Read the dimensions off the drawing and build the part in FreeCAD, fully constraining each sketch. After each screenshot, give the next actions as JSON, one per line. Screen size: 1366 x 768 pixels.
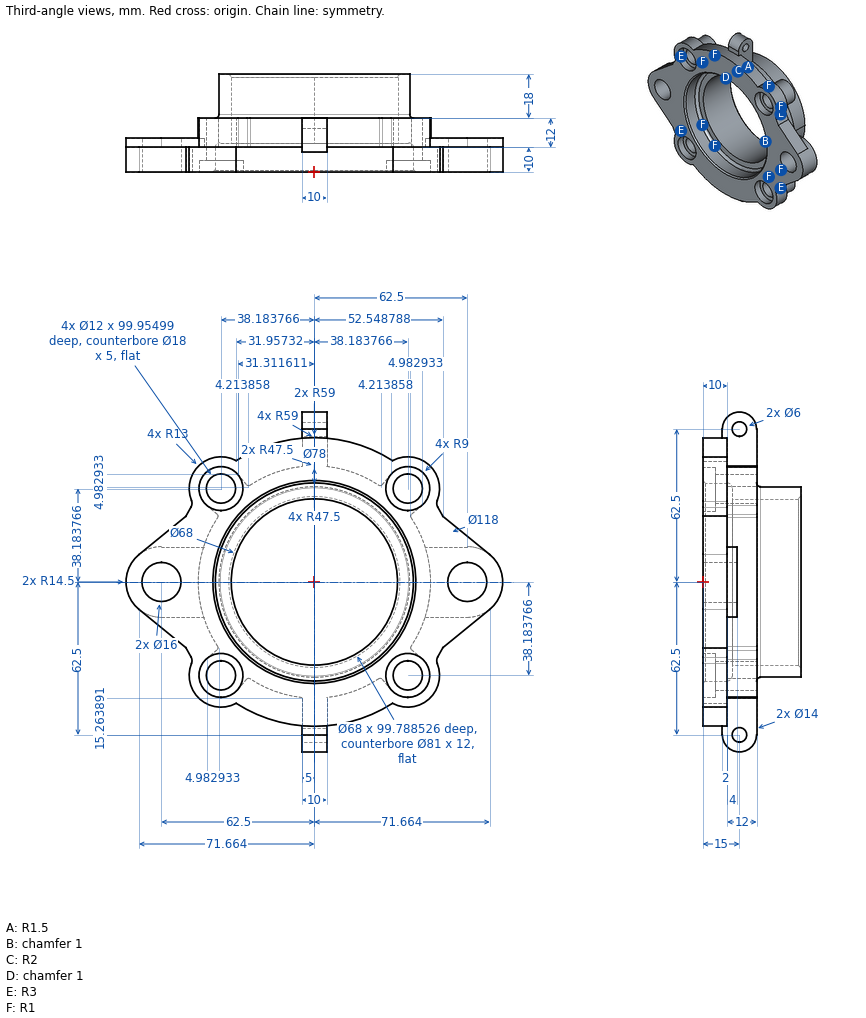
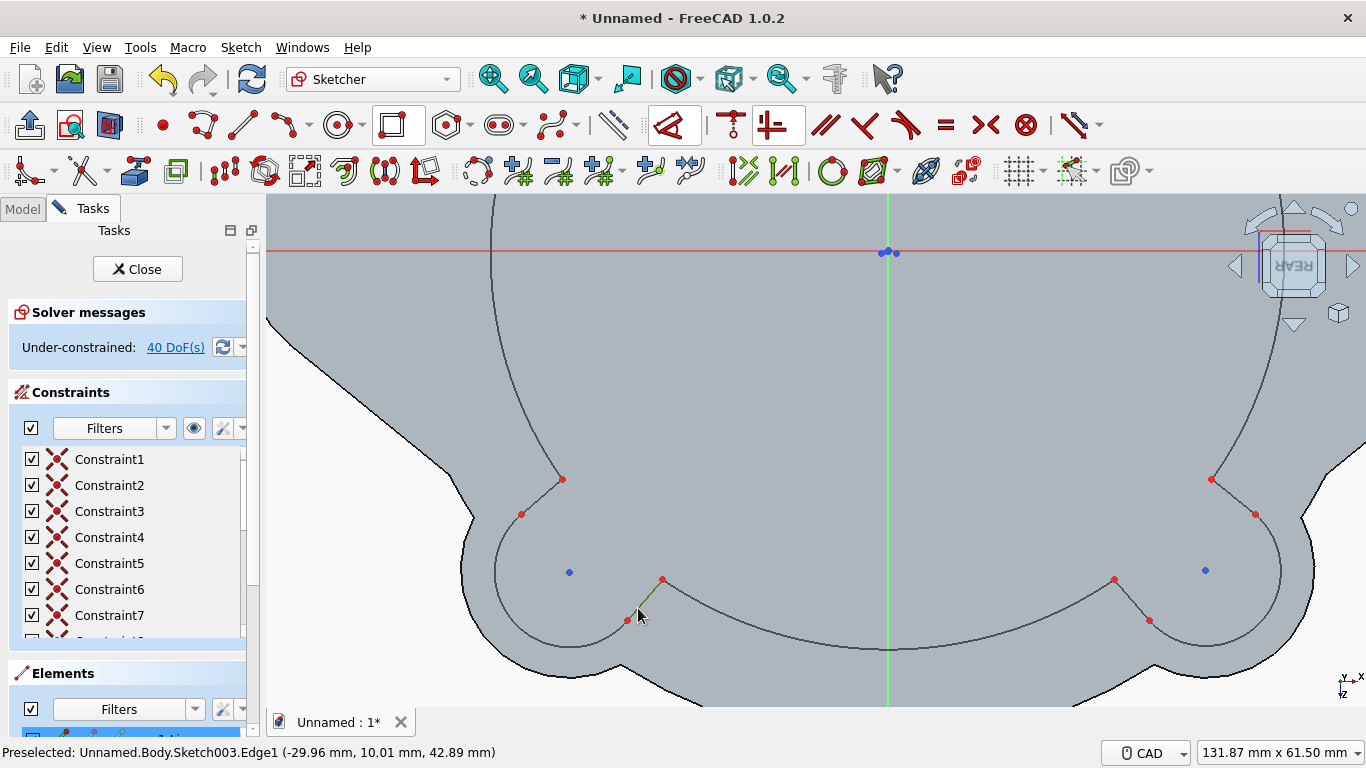
{"action": "left_click", "coordinate": [495, 581]}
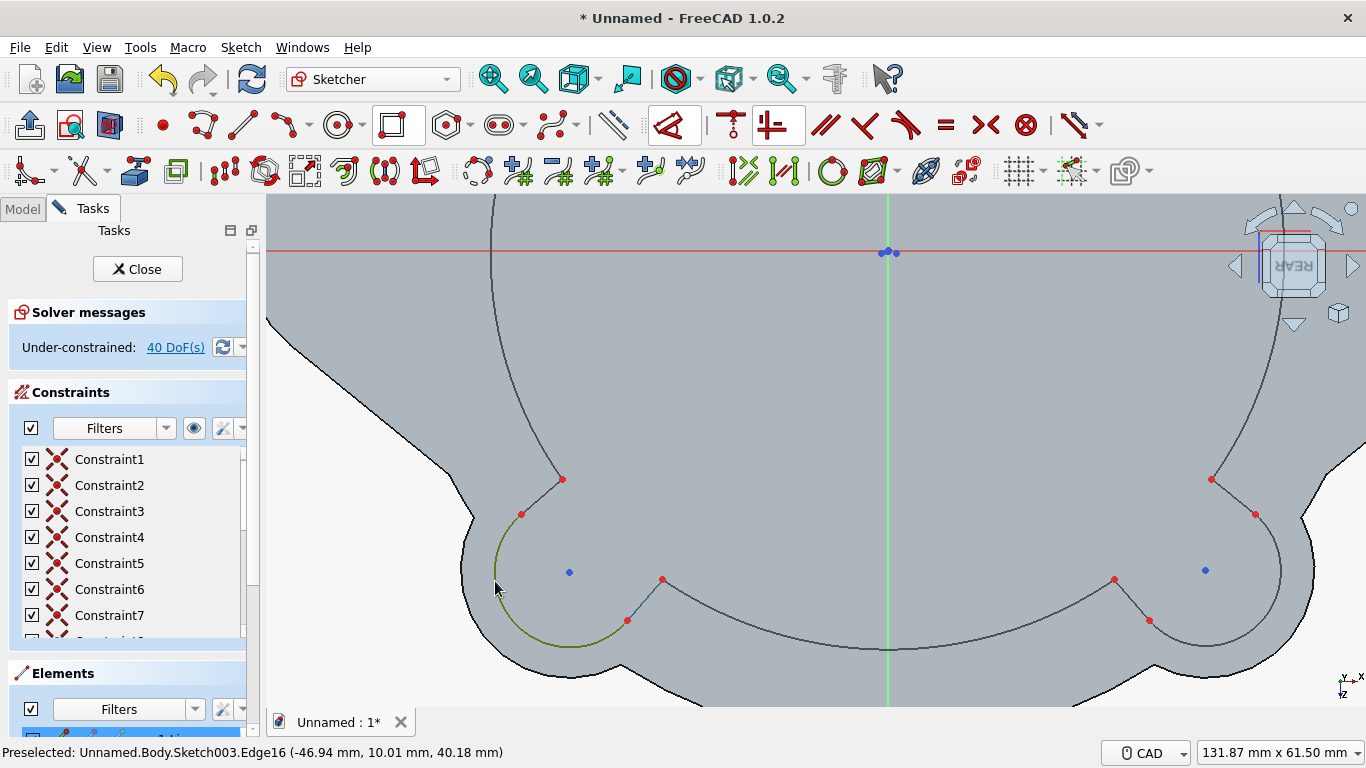
{"action": "left_click", "coordinate": [906, 126]}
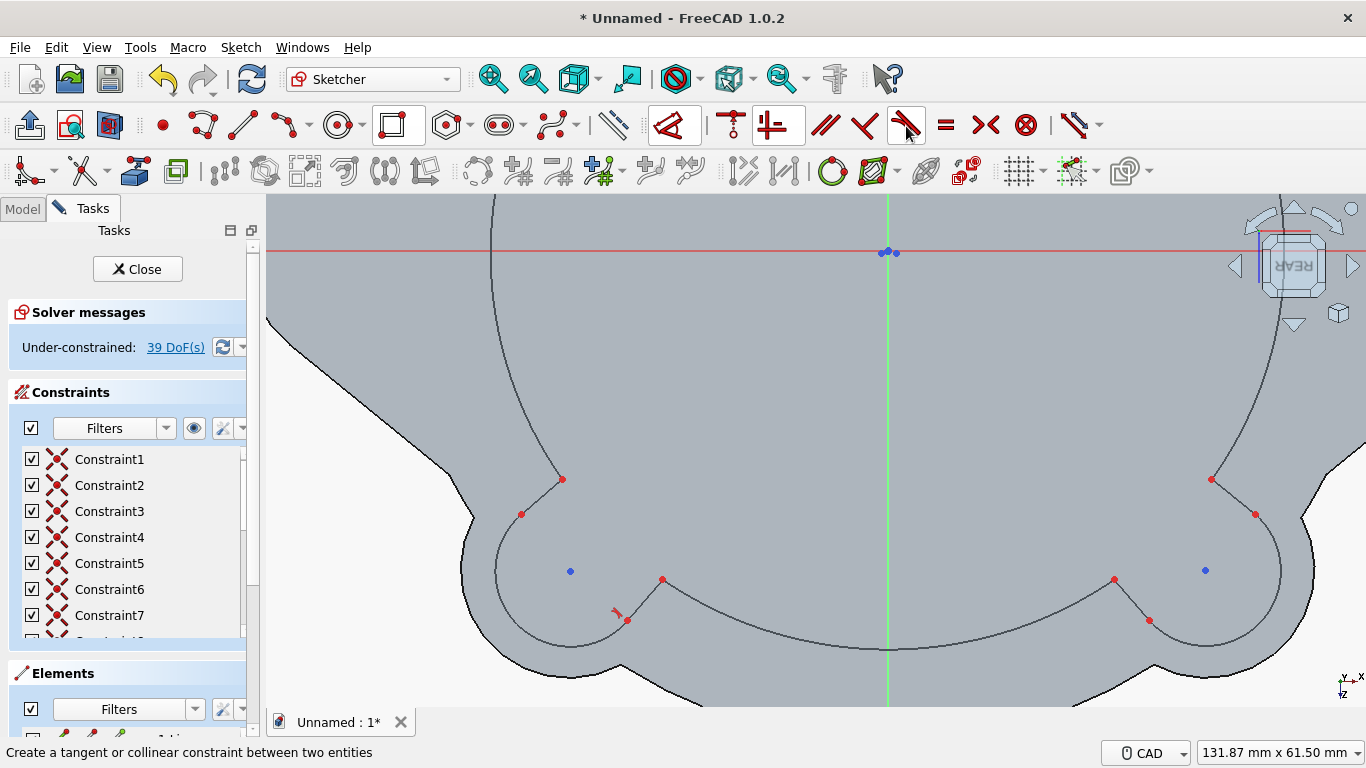
{"action": "left_click", "coordinate": [1125, 592]}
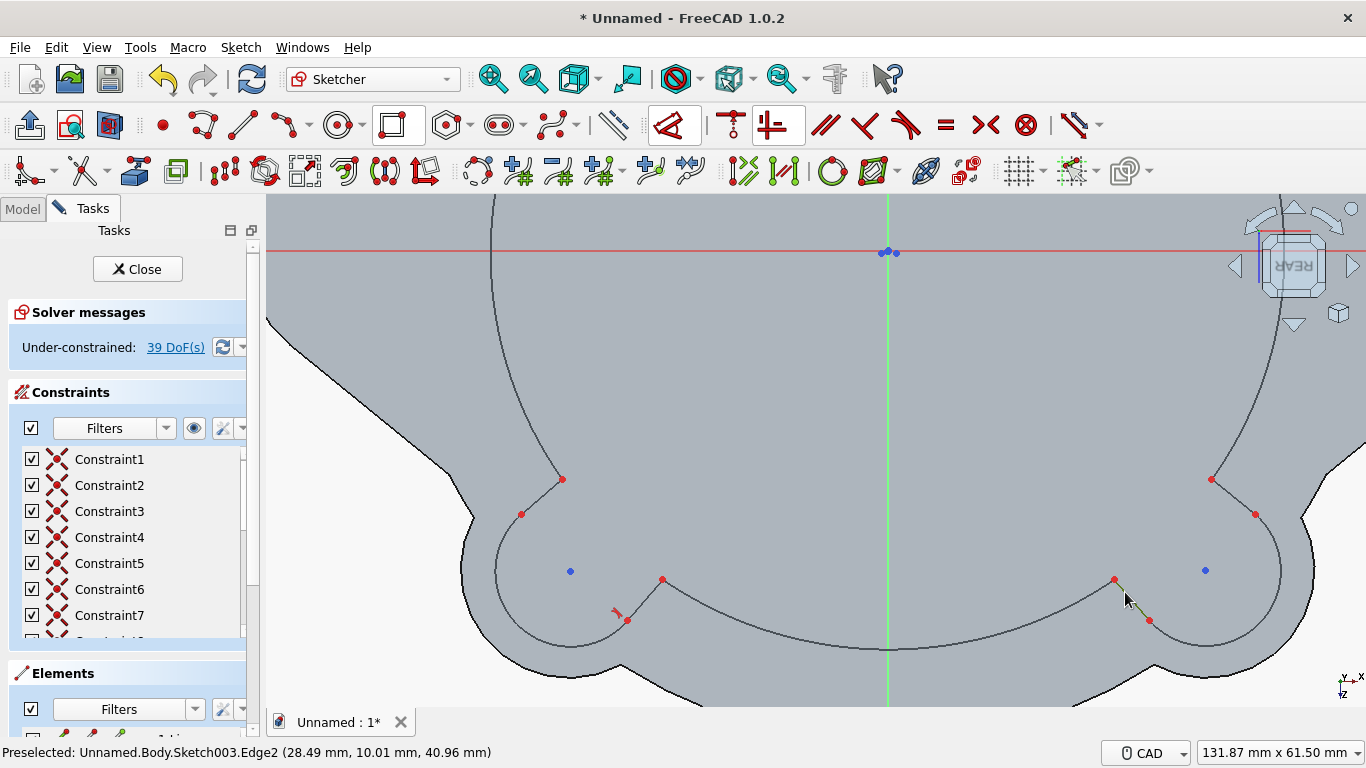
{"action": "left_click", "coordinate": [1191, 645]}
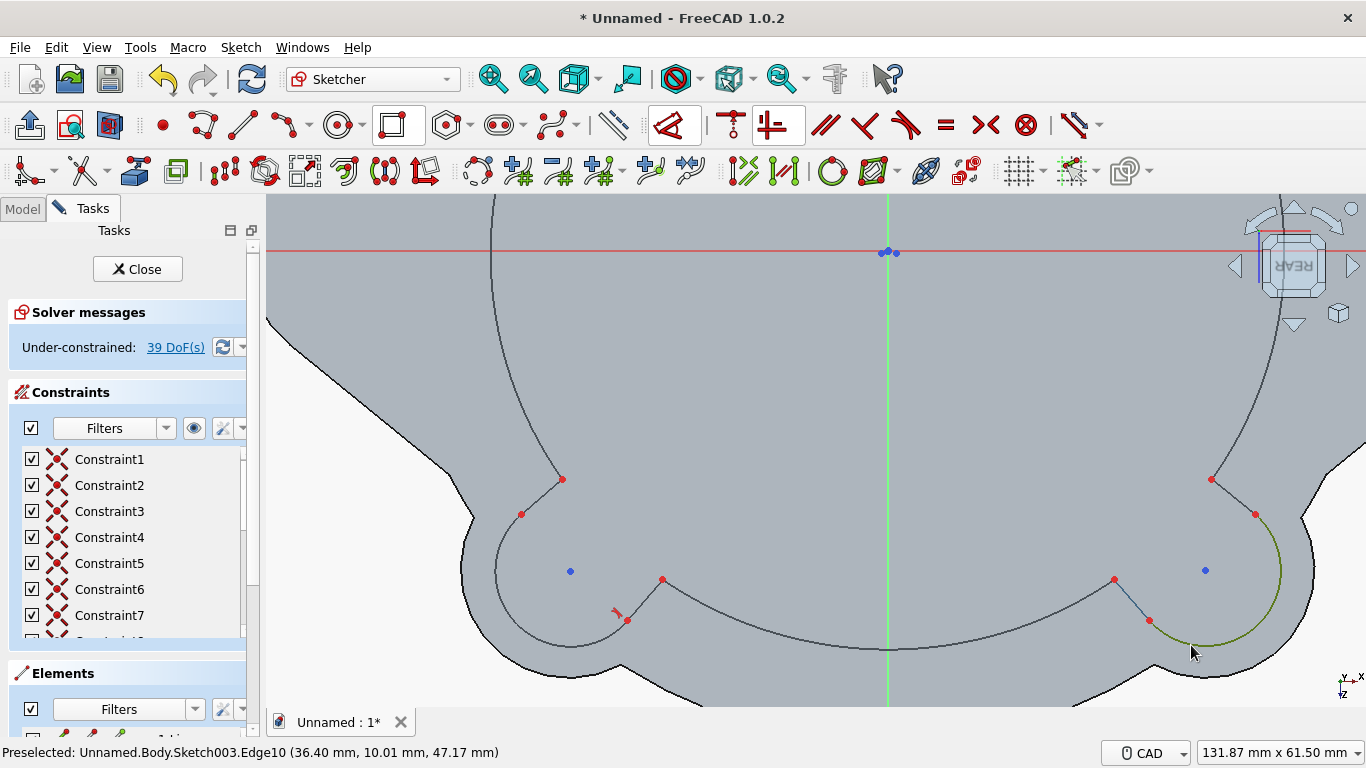
{"action": "left_click", "coordinate": [906, 126]}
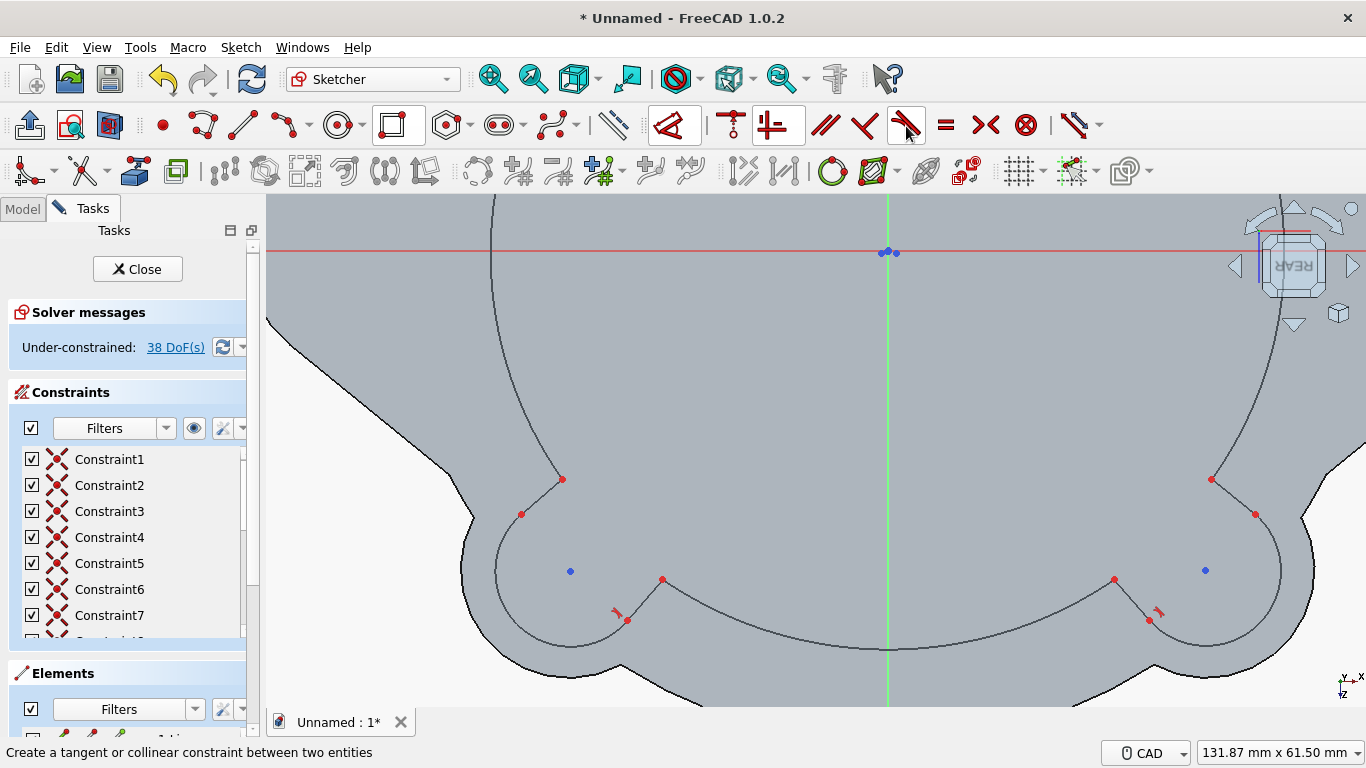
{"action": "scroll", "coordinate": [633, 613], "scroll_direction": "down", "scroll_amount": 4}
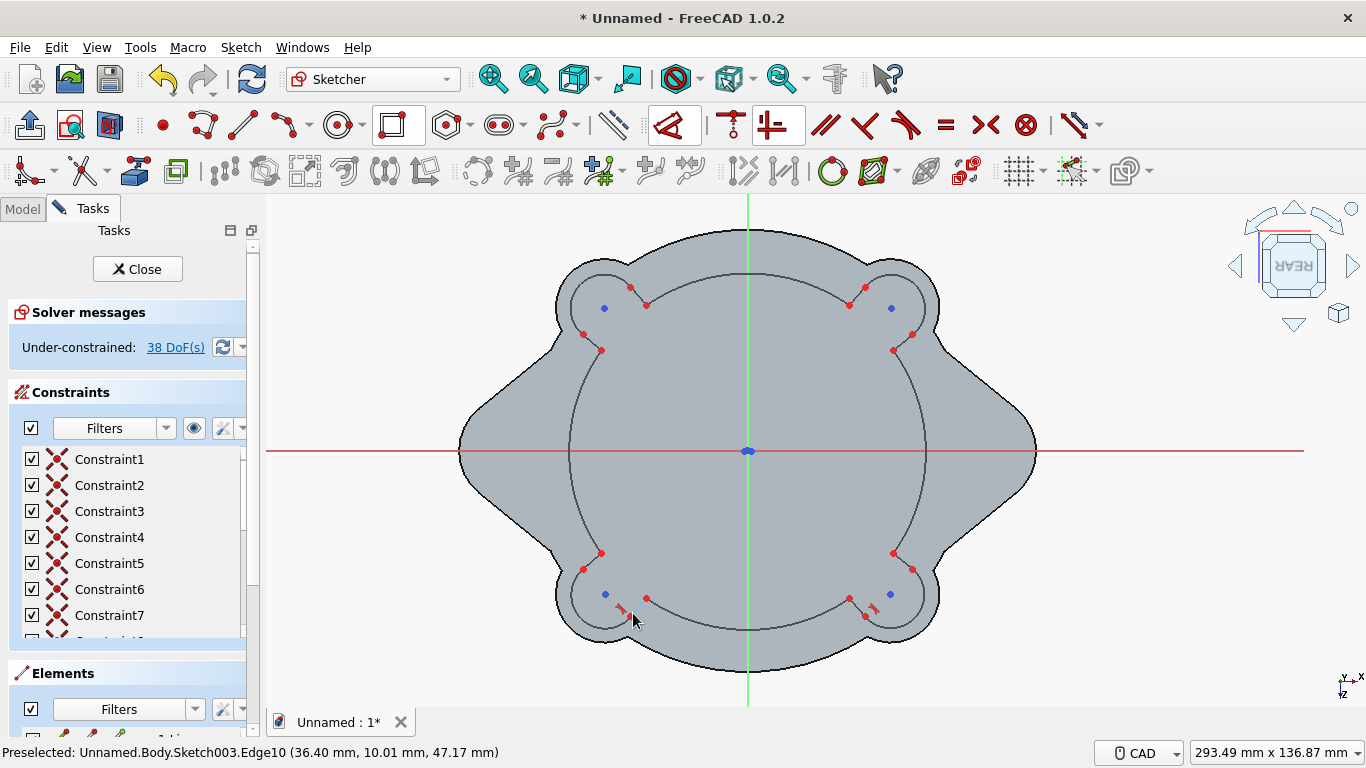
{"action": "scroll", "coordinate": [907, 564], "scroll_direction": "up", "scroll_amount": 4}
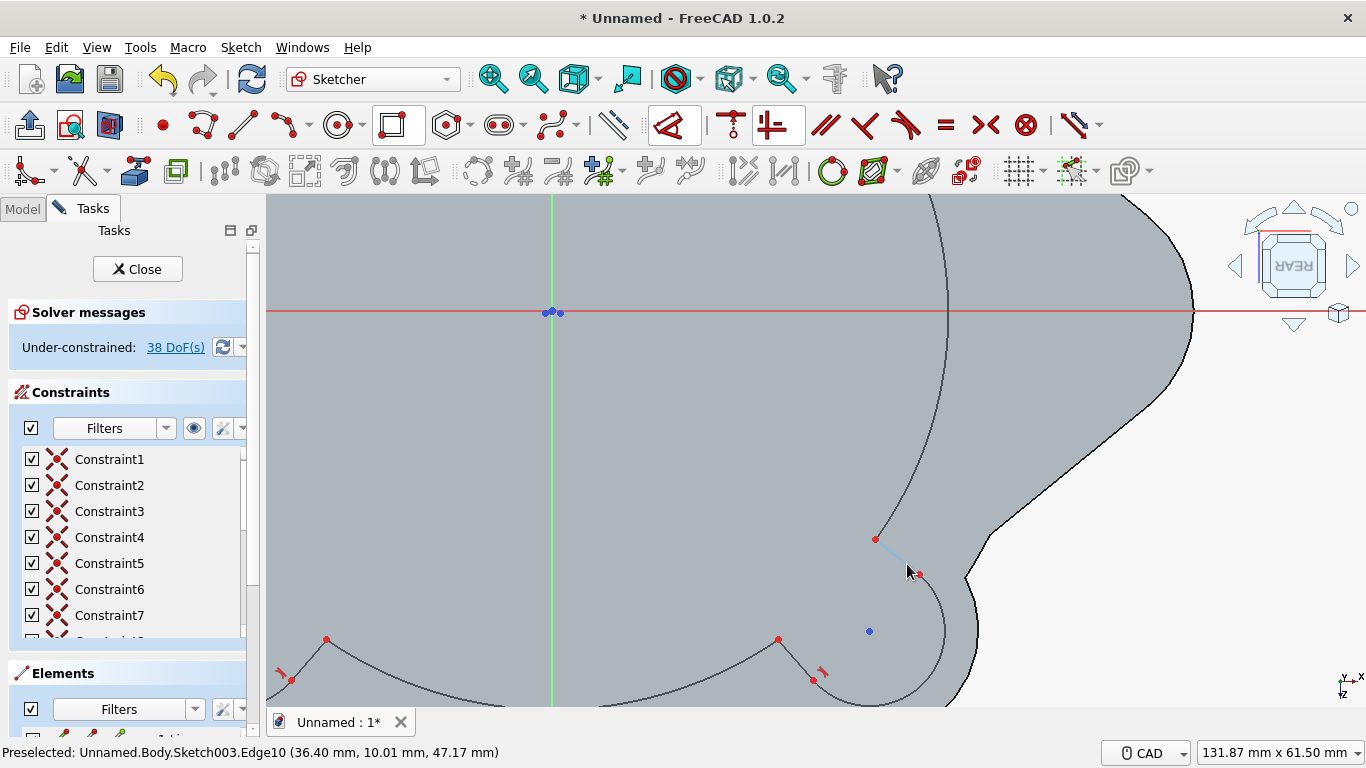
{"action": "left_click", "coordinate": [906, 564]}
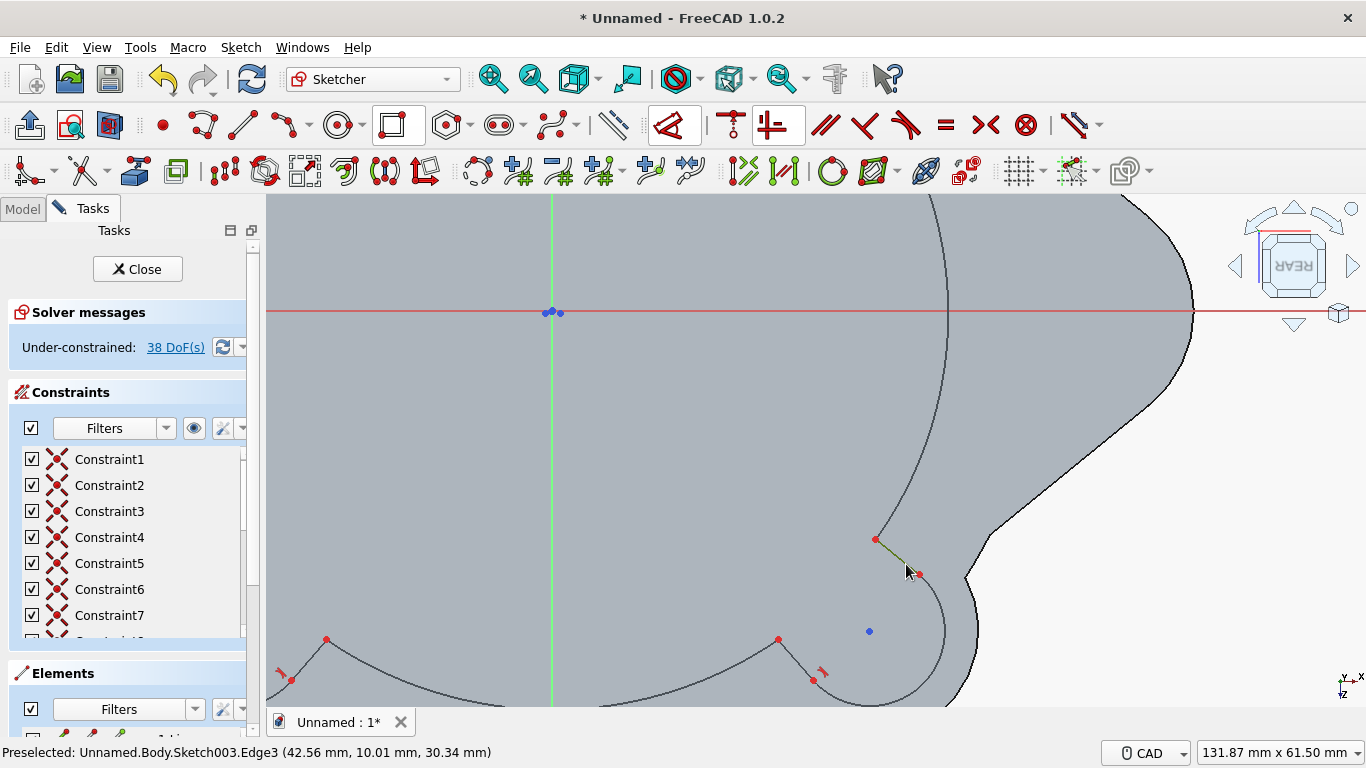
{"action": "left_click", "coordinate": [944, 641]}